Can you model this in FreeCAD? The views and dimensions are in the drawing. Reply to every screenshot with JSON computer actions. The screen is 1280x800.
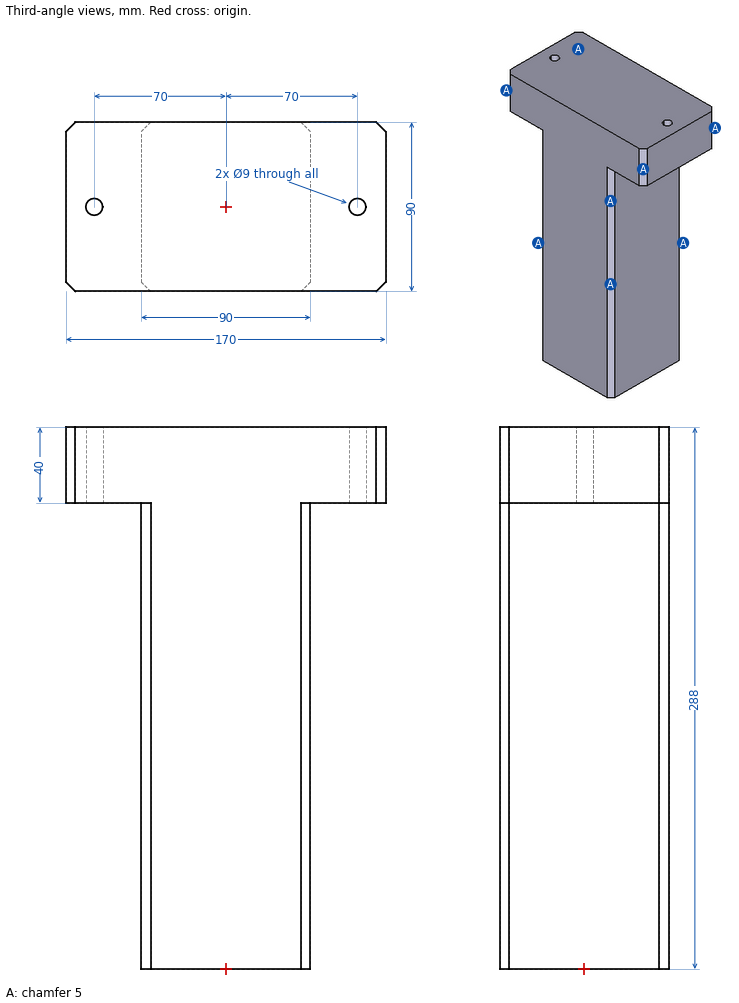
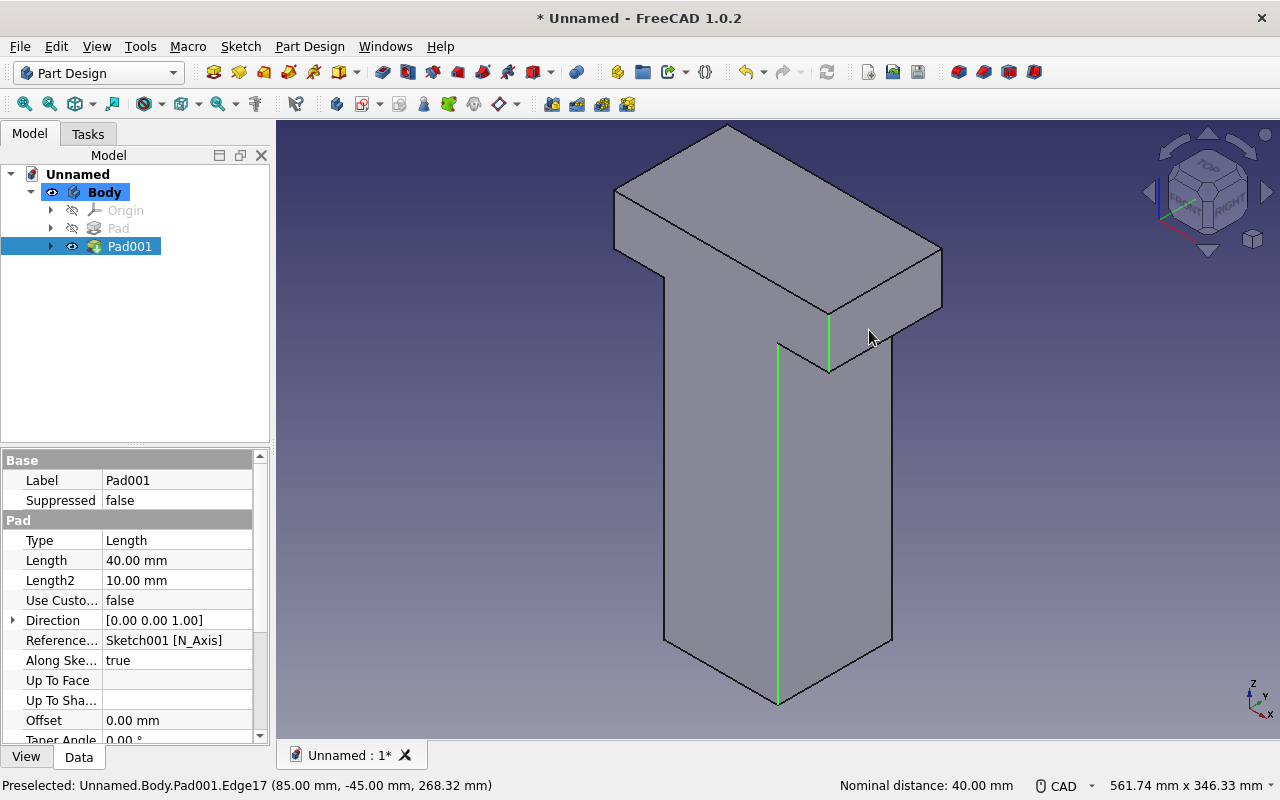
{"action": "key", "text": "2"}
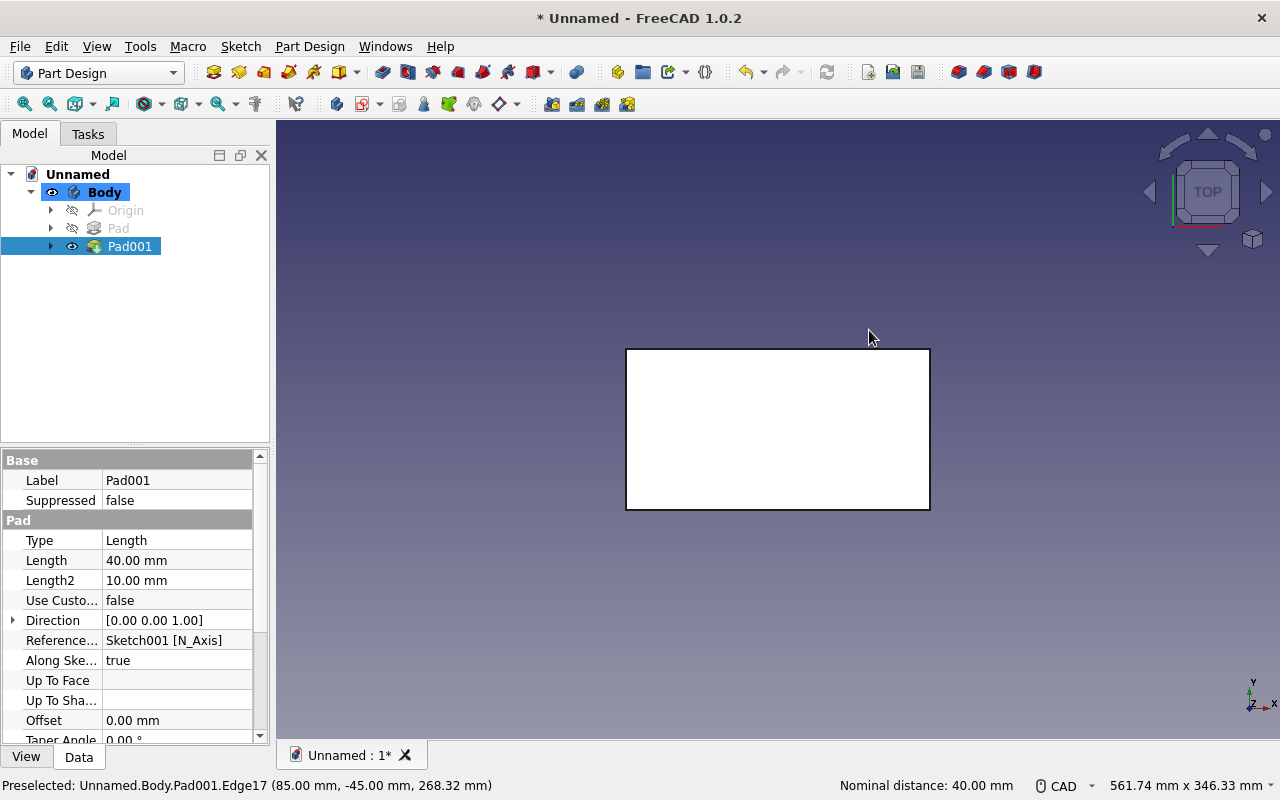
{"action": "left_click", "coordinate": [25, 104]}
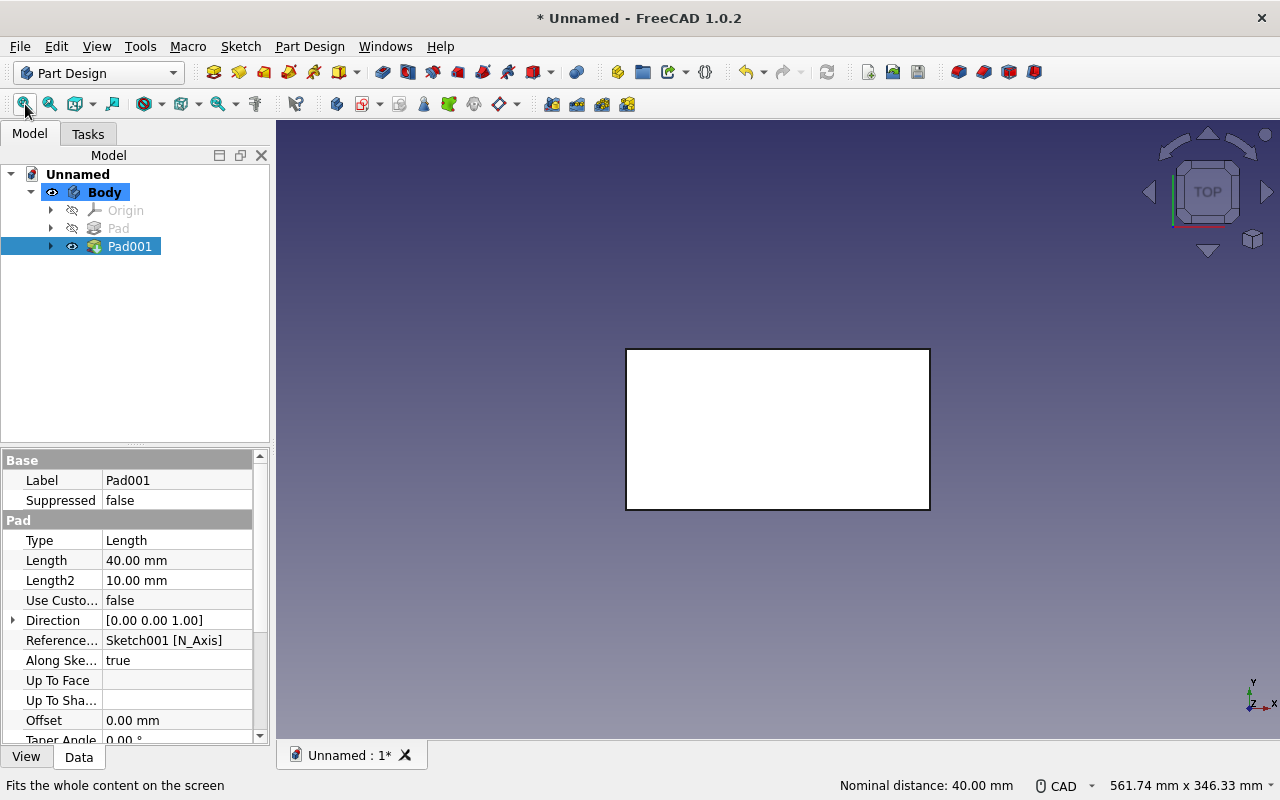
{"action": "key", "text": "1"}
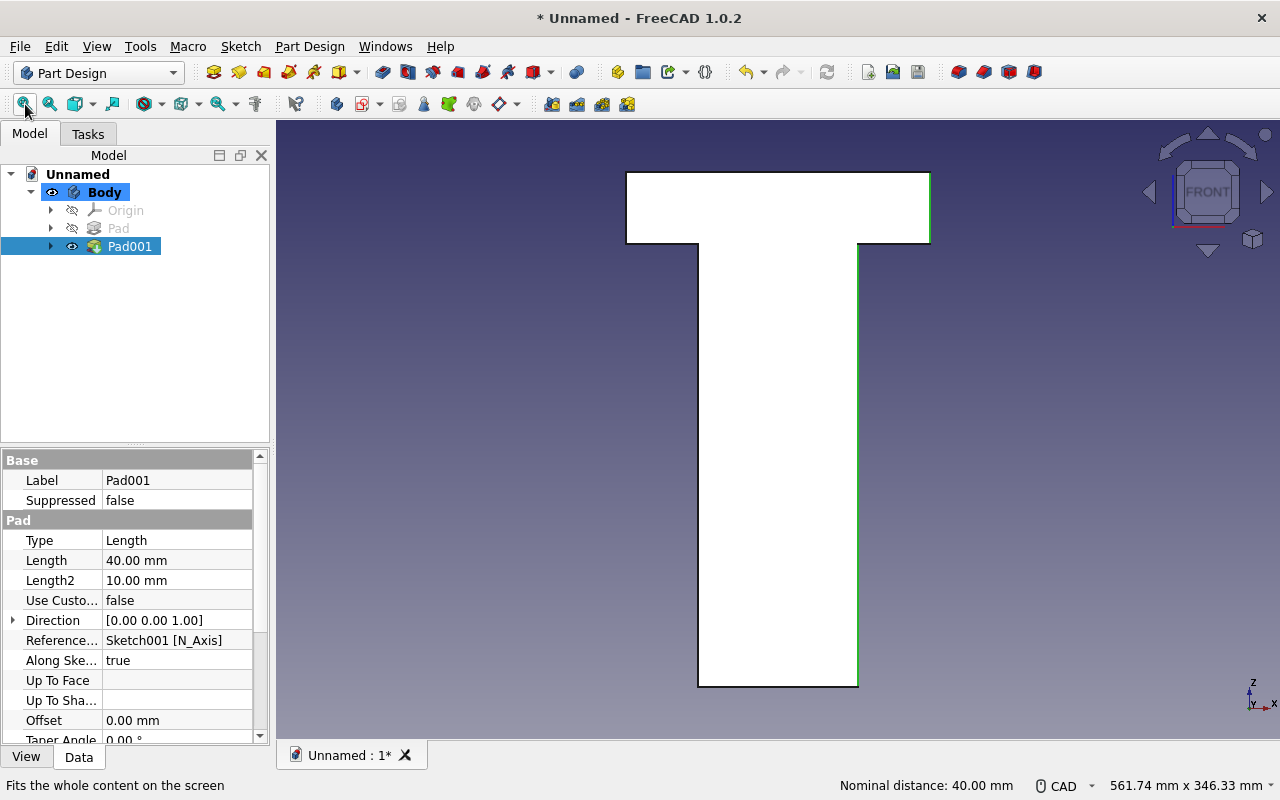
{"action": "left_click", "coordinate": [698, 464], "text": "ctrl"}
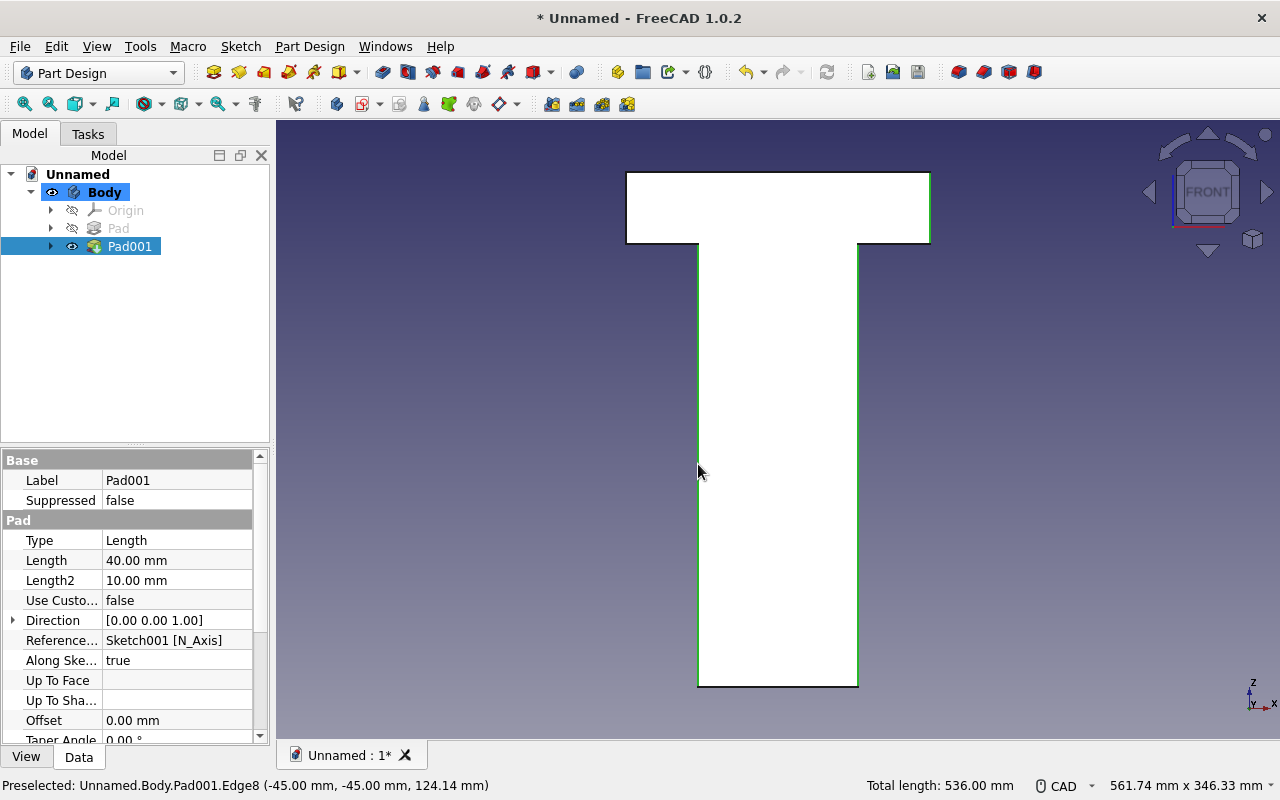
{"action": "left_click", "coordinate": [626, 207], "text": "ctrl"}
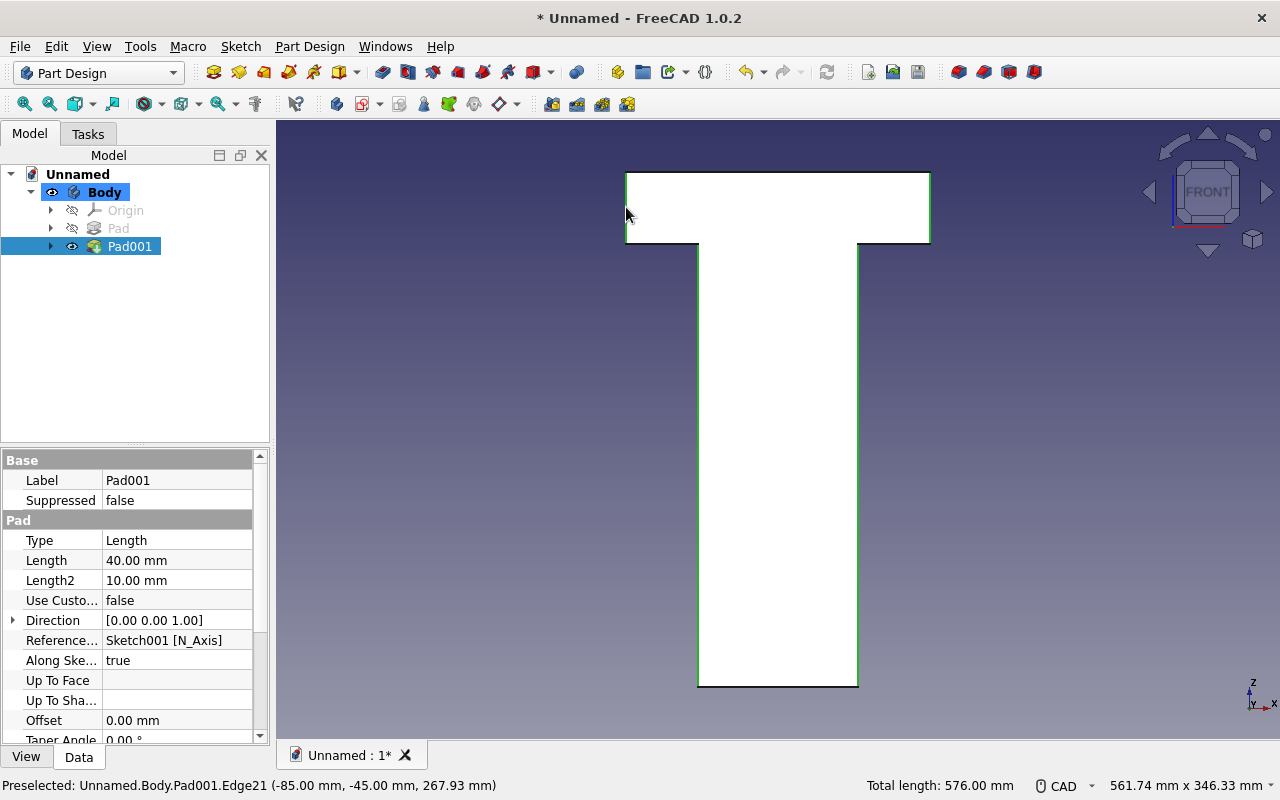
{"action": "key", "text": "3"}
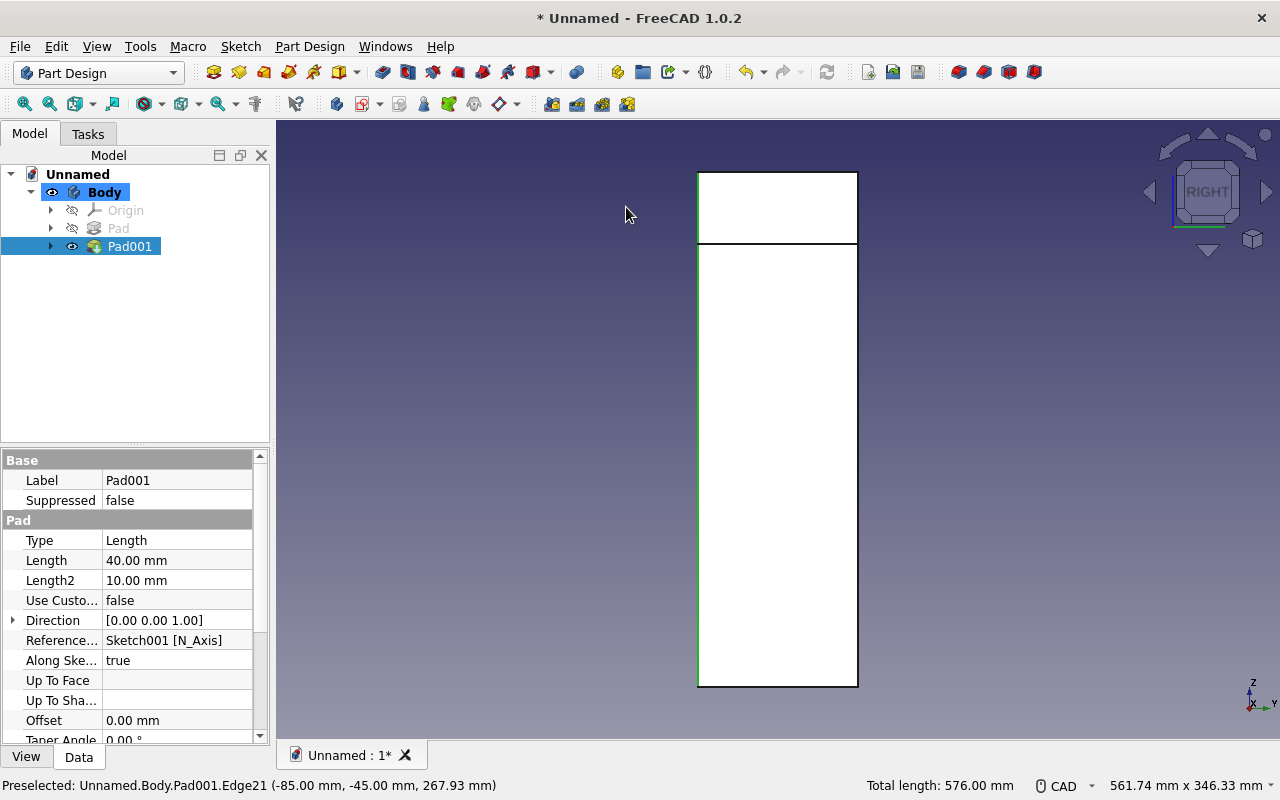
{"action": "left_click", "coordinate": [858, 464], "text": "ctrl"}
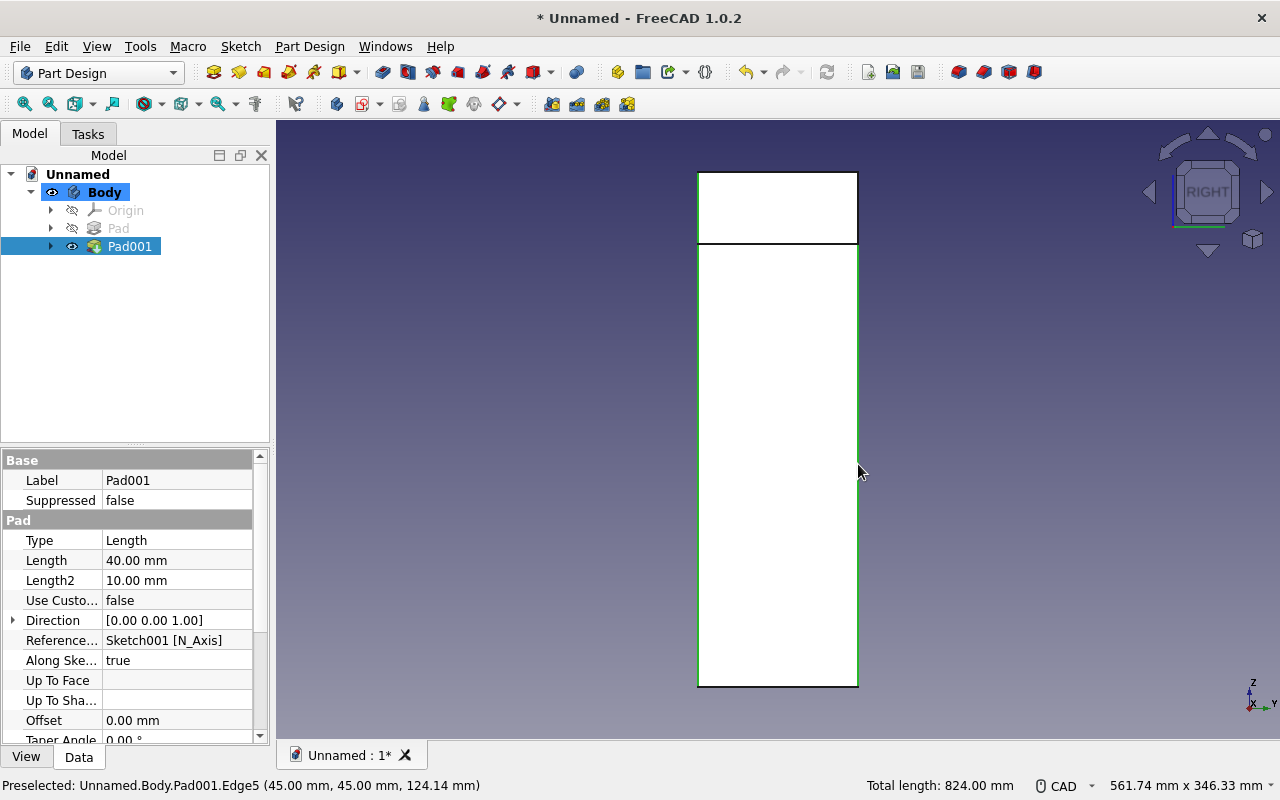
{"action": "left_click", "coordinate": [858, 207], "text": "ctrl"}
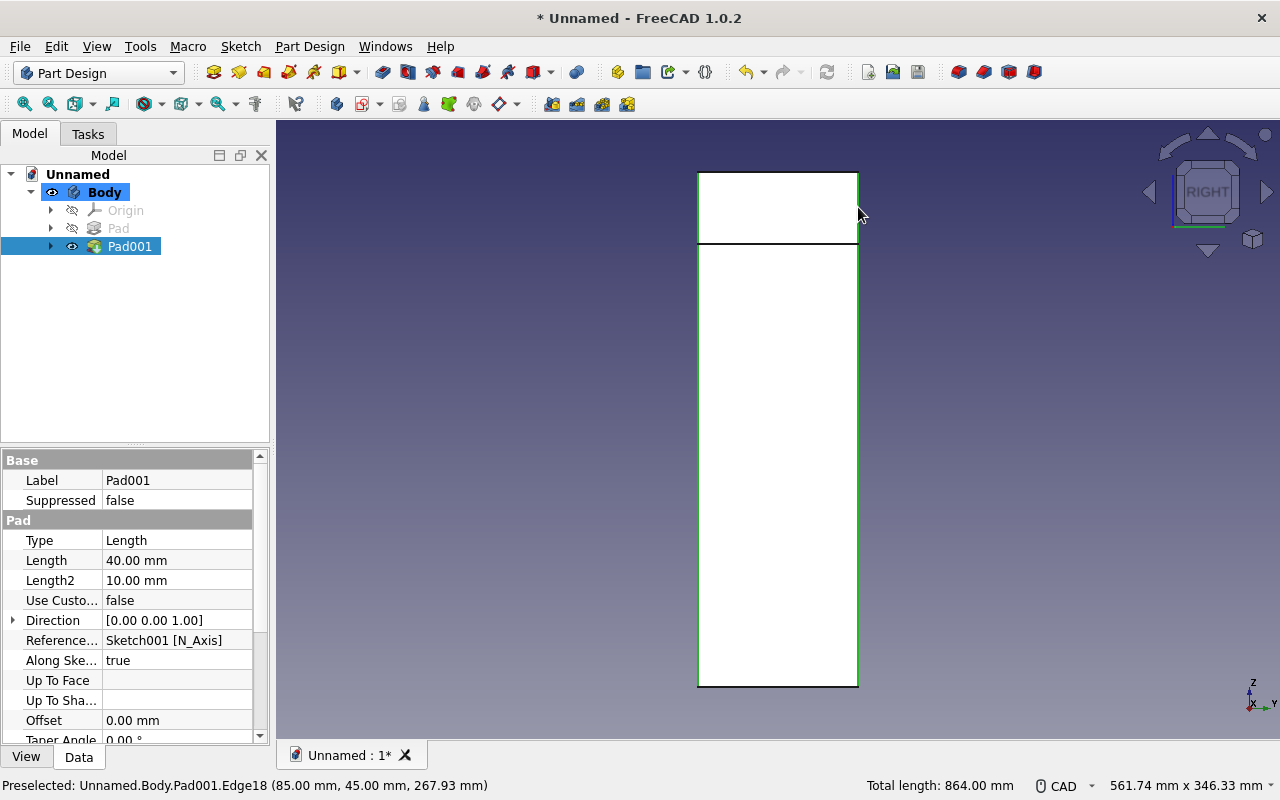
{"action": "key", "text": "5"}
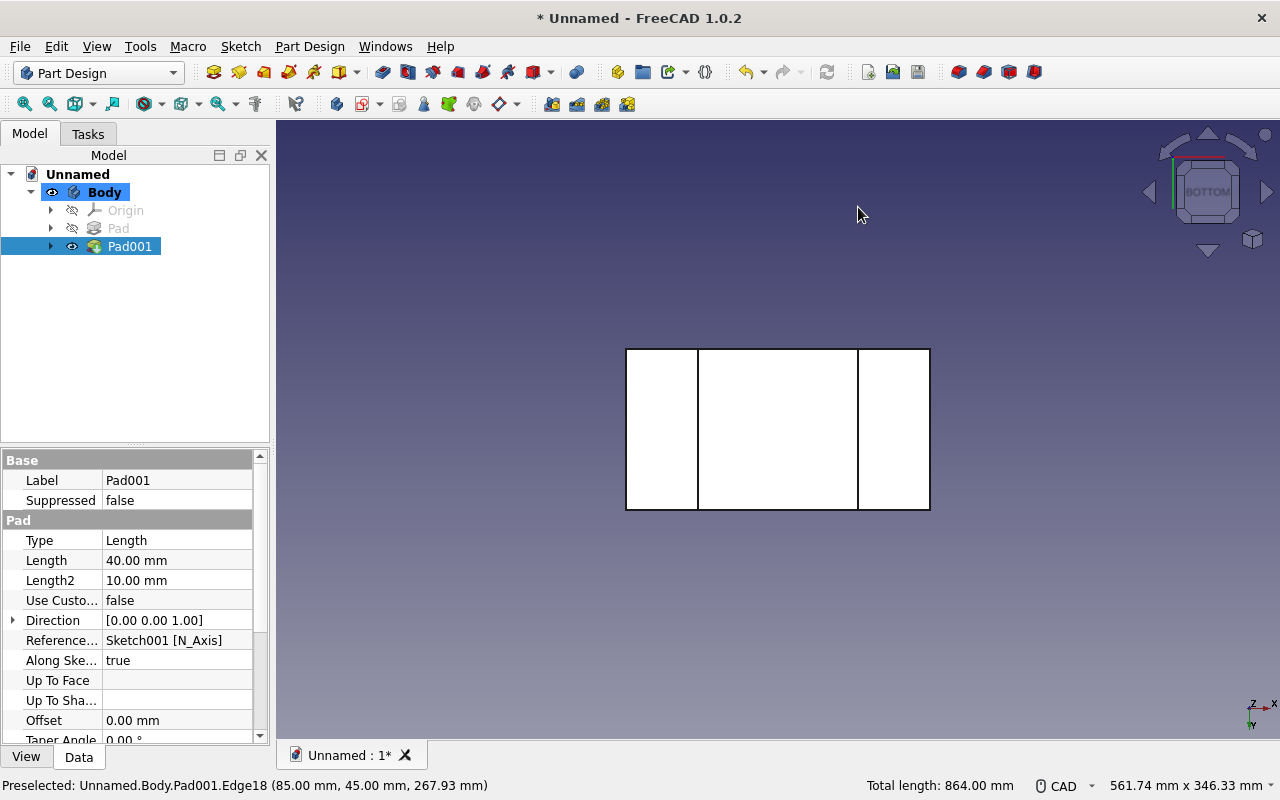
{"action": "left_click", "coordinate": [25, 104]}